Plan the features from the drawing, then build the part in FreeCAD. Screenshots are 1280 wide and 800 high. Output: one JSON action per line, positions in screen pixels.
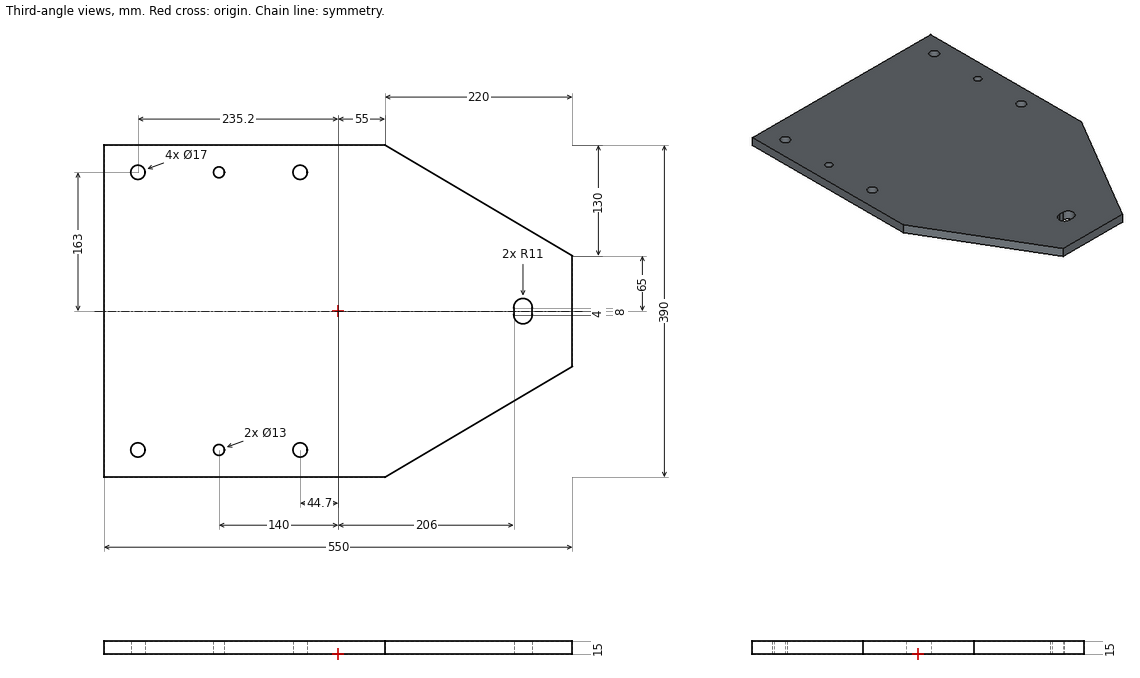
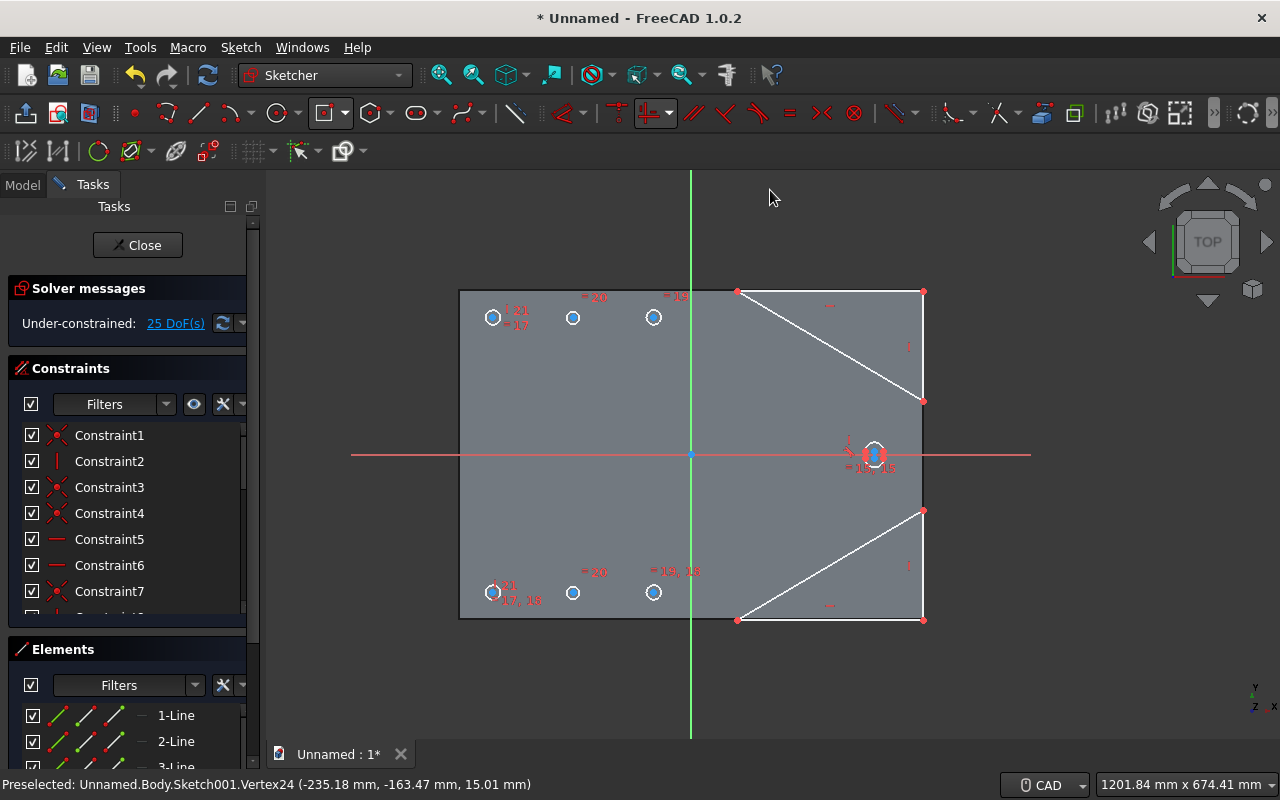
{"action": "scroll", "coordinate": [493, 593], "scroll_direction": "up", "scroll_amount": 4}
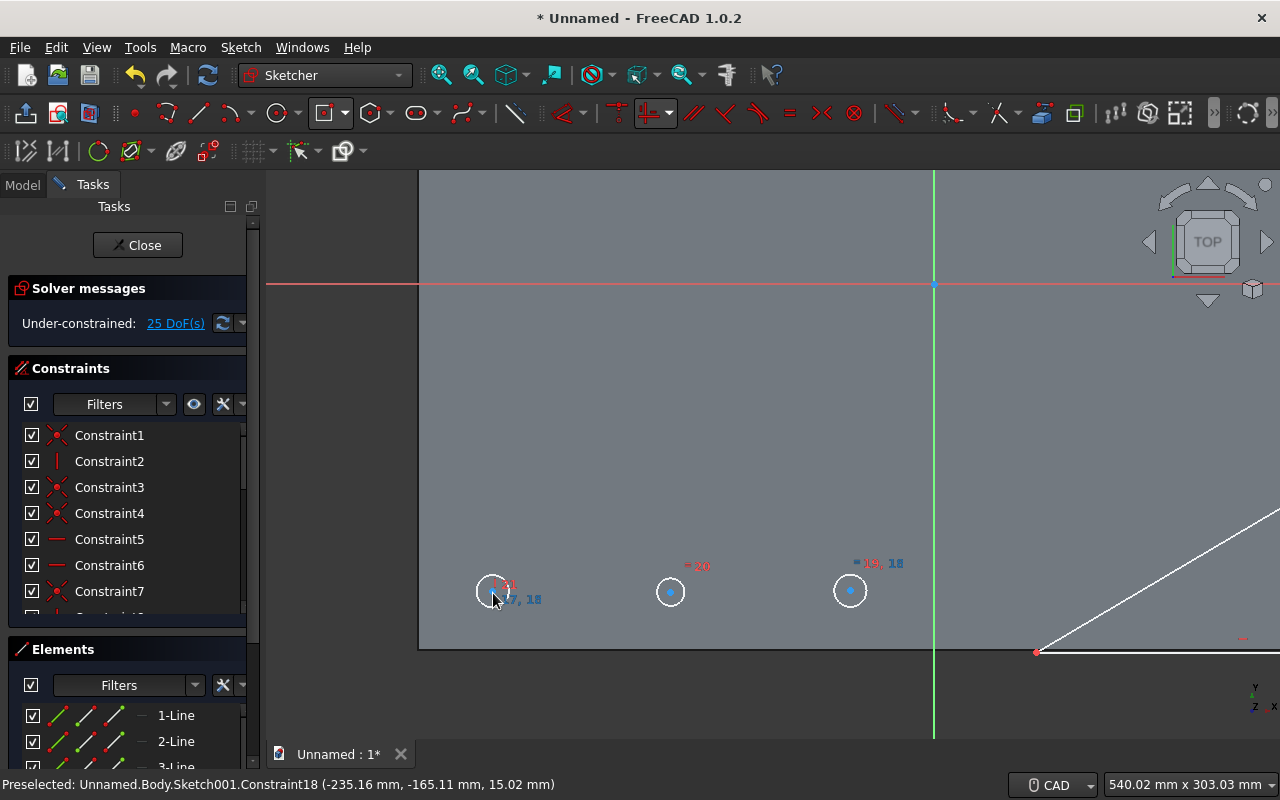
{"action": "scroll", "coordinate": [493, 591], "scroll_direction": "up", "scroll_amount": 4}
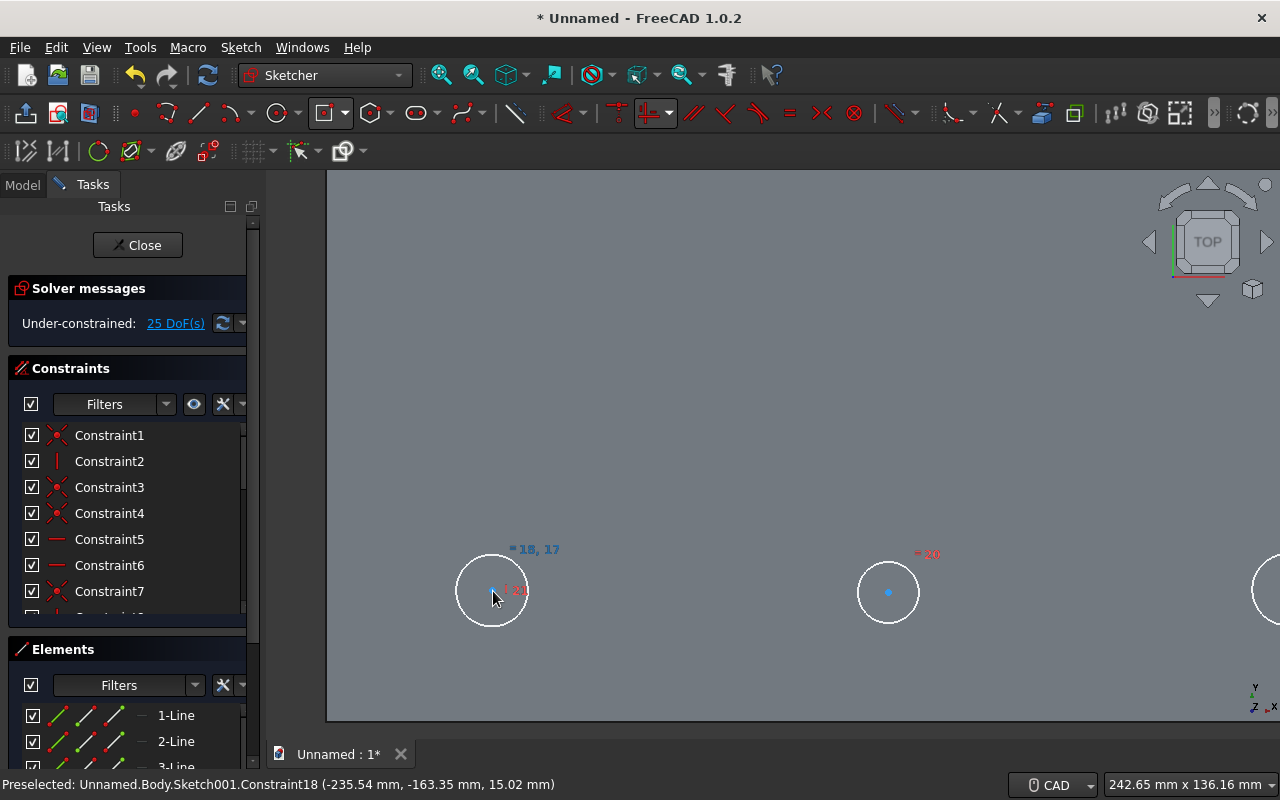
{"action": "left_click", "coordinate": [492, 591]}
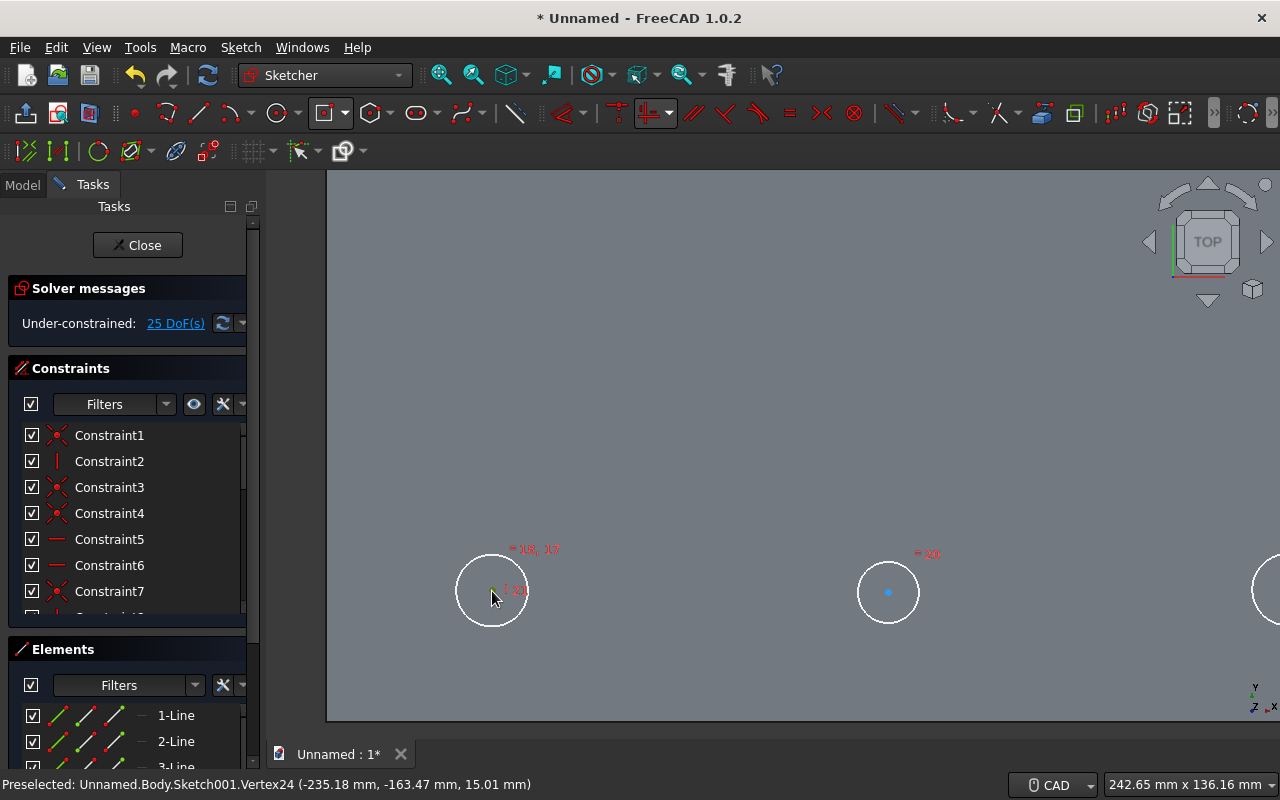
{"action": "scroll", "coordinate": [493, 593], "scroll_direction": "down", "scroll_amount": 8}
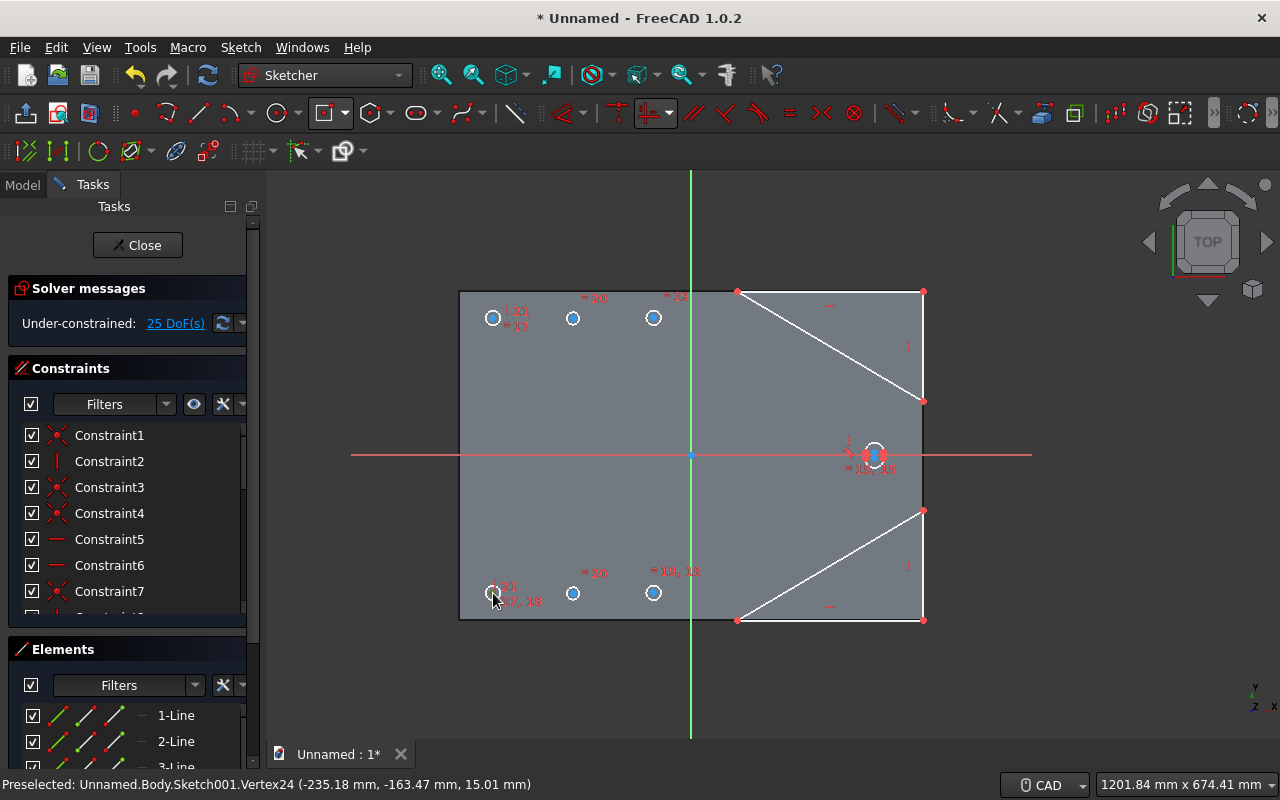
{"action": "left_click", "coordinate": [573, 593]}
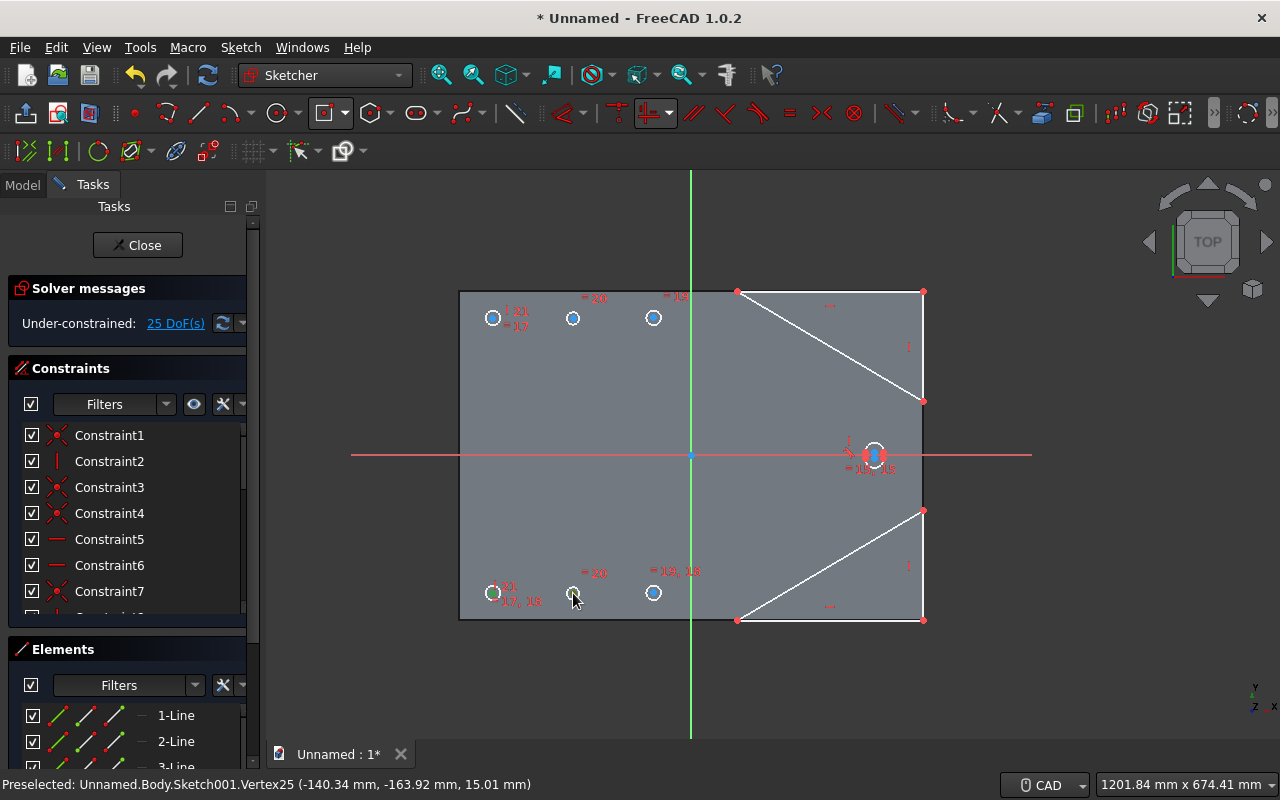
{"action": "key", "text": "h"}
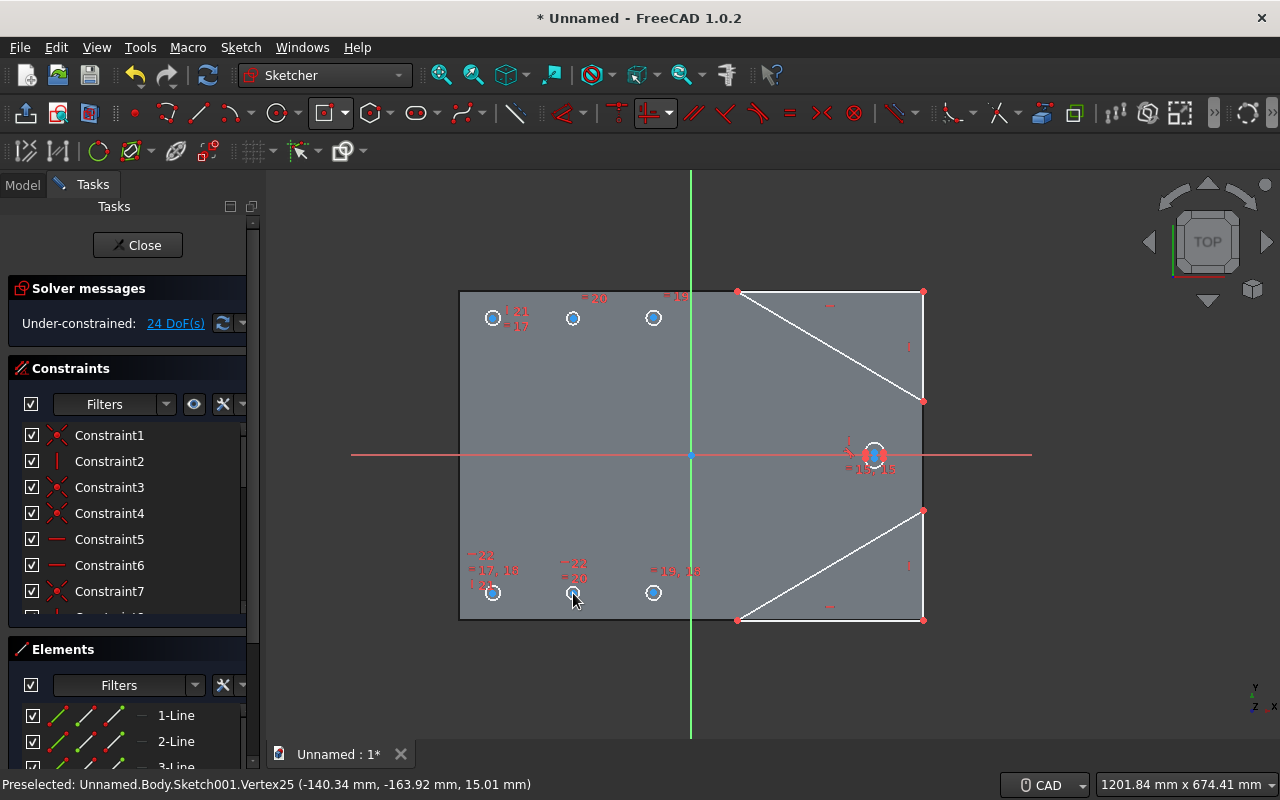
{"action": "left_click", "coordinate": [573, 593]}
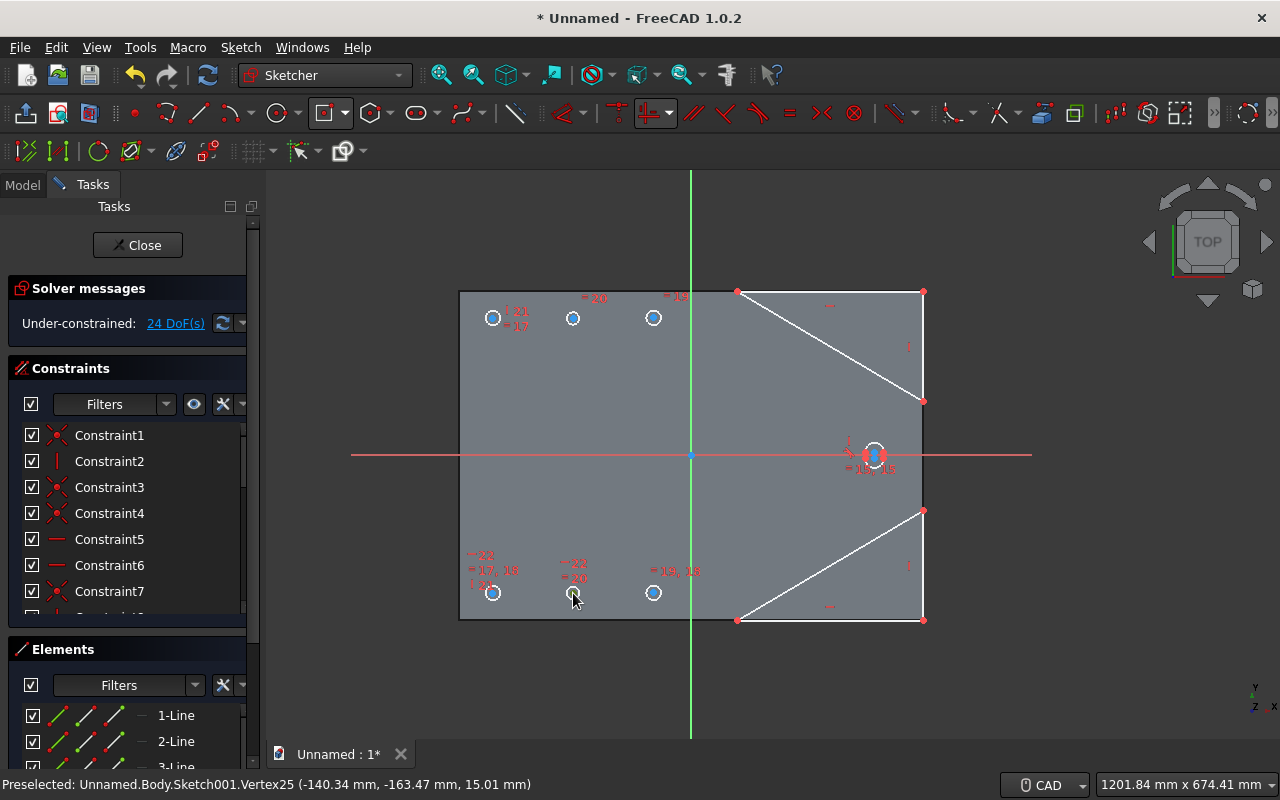
{"action": "left_click", "coordinate": [654, 593]}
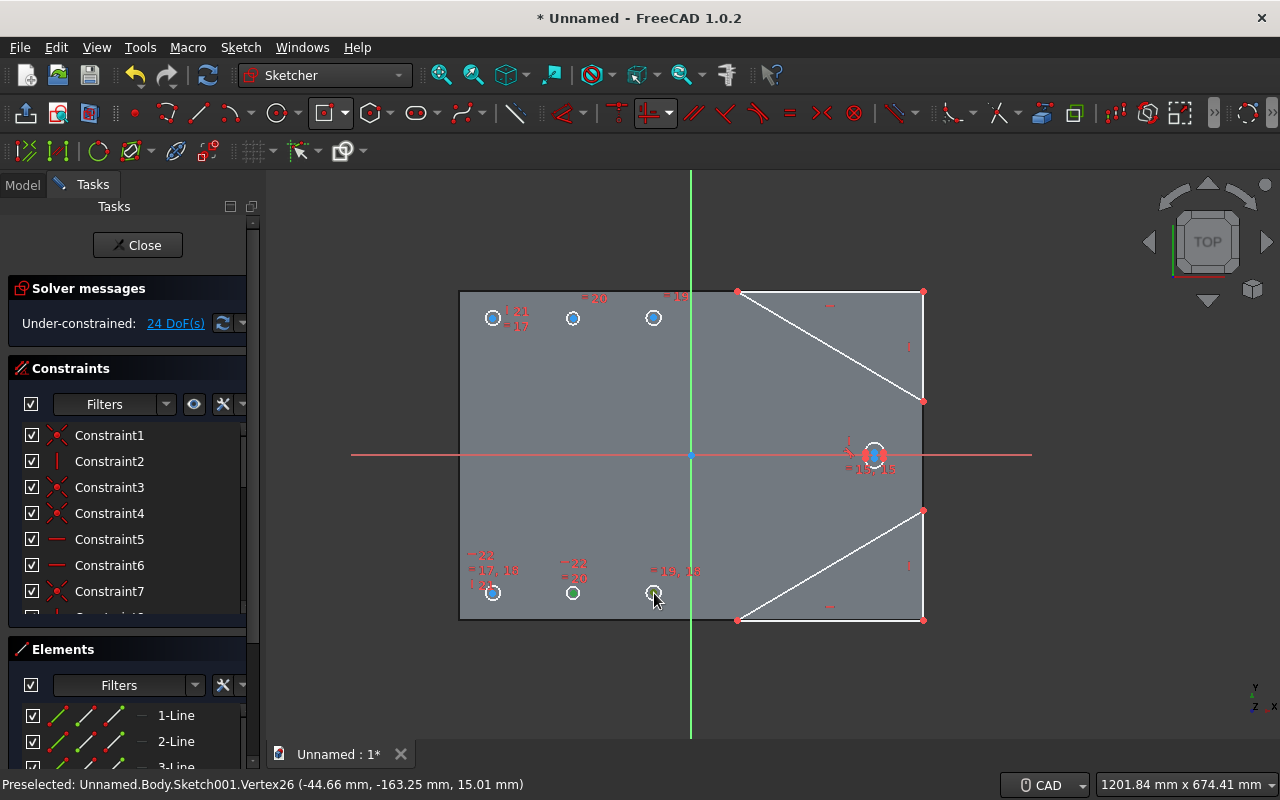
{"action": "left_click", "coordinate": [672, 114]}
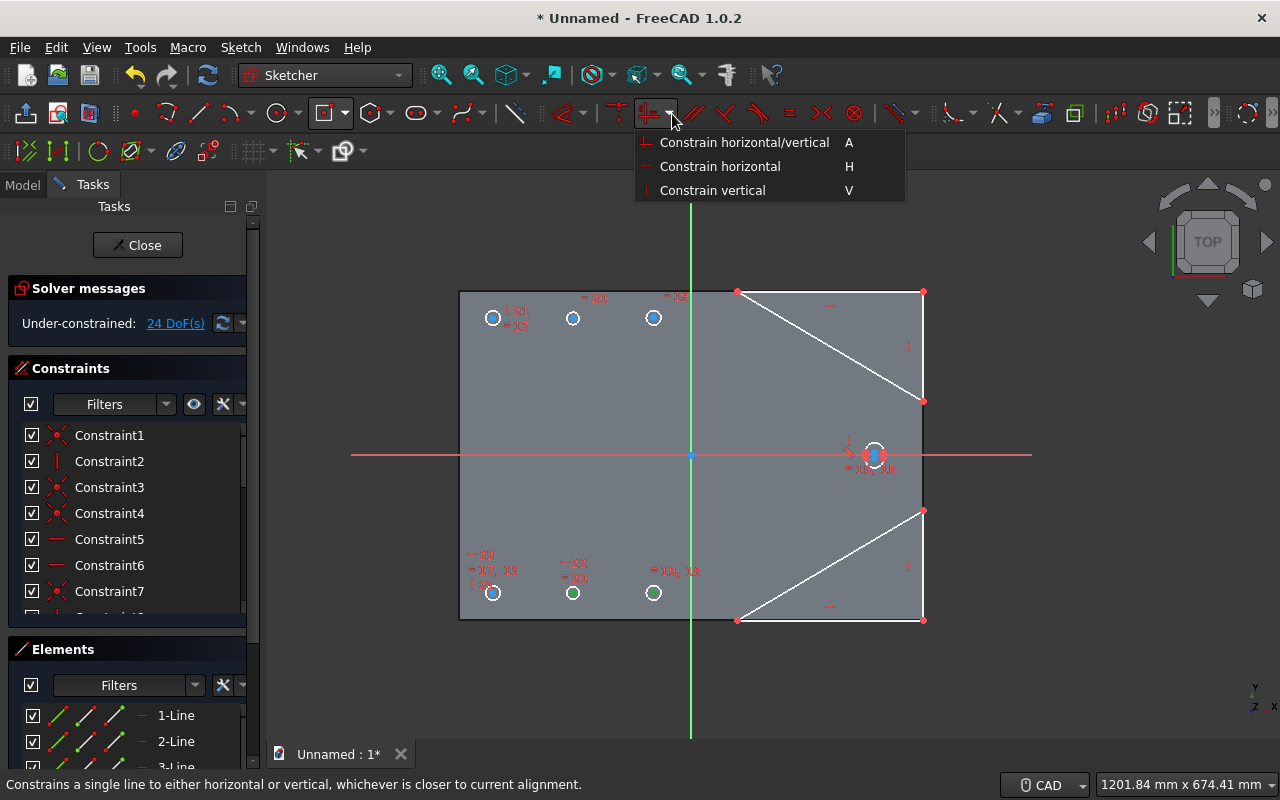
{"action": "left_click", "coordinate": [770, 166]}